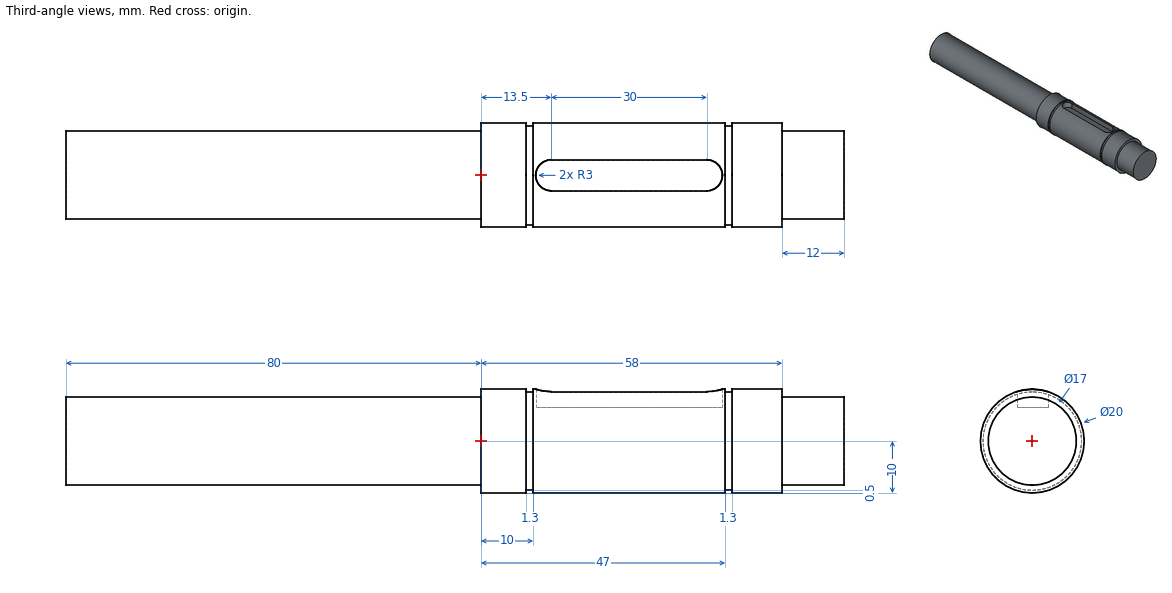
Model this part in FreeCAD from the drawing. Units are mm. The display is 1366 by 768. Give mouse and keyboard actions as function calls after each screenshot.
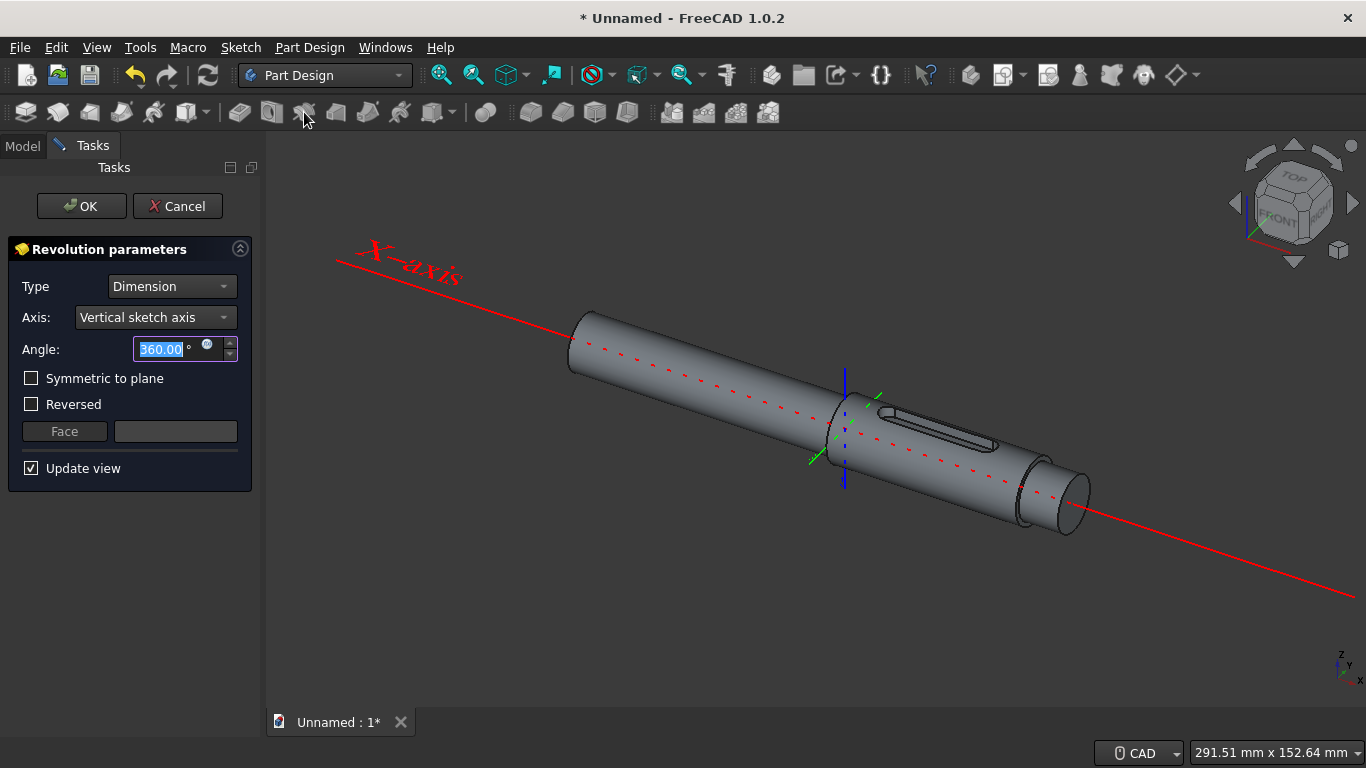
click(156, 318)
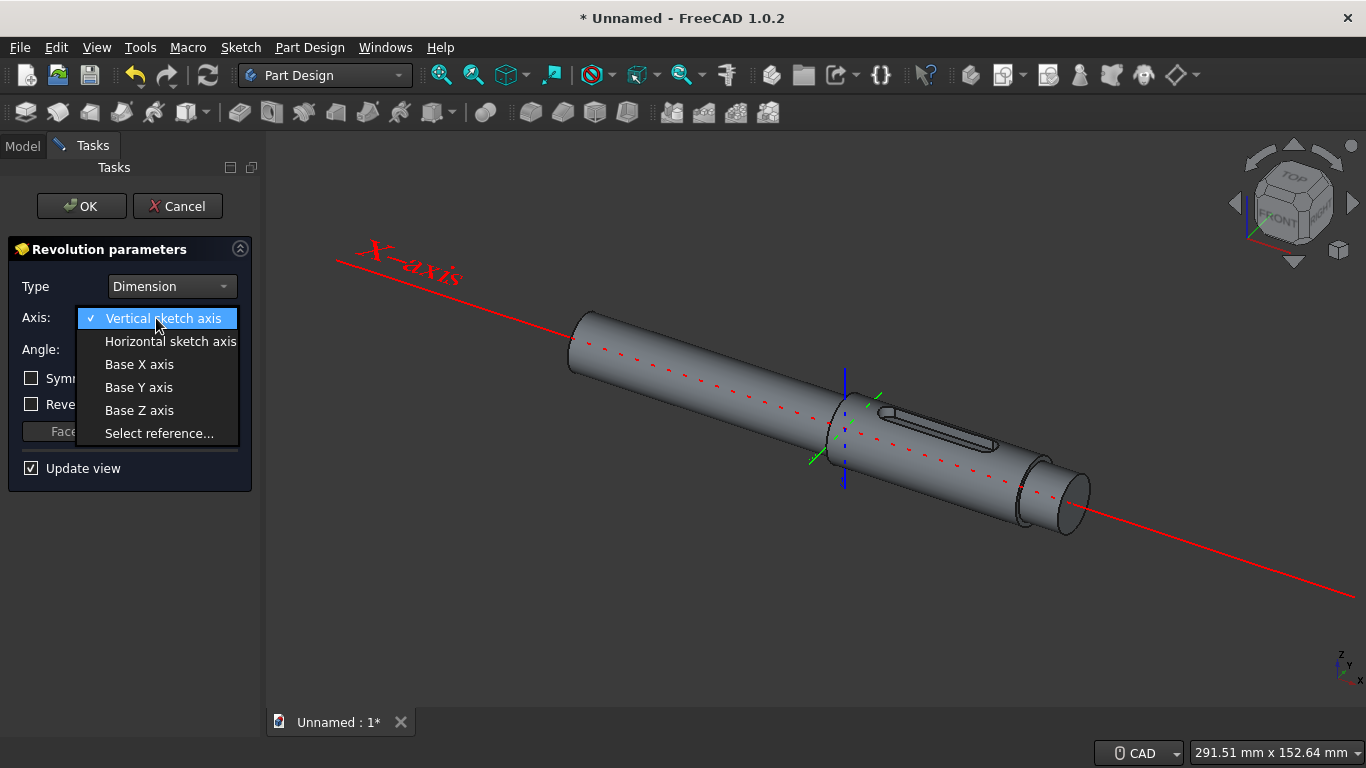
click(156, 342)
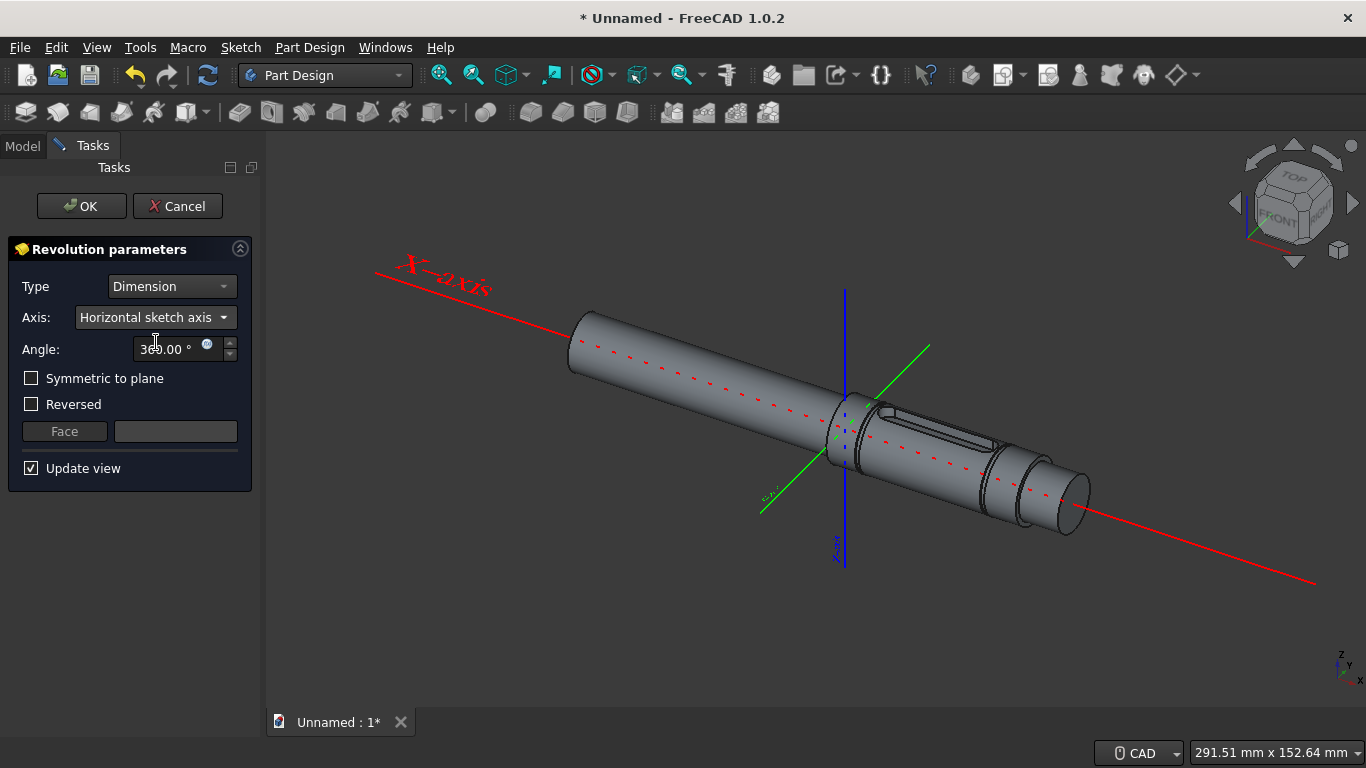
click(82, 206)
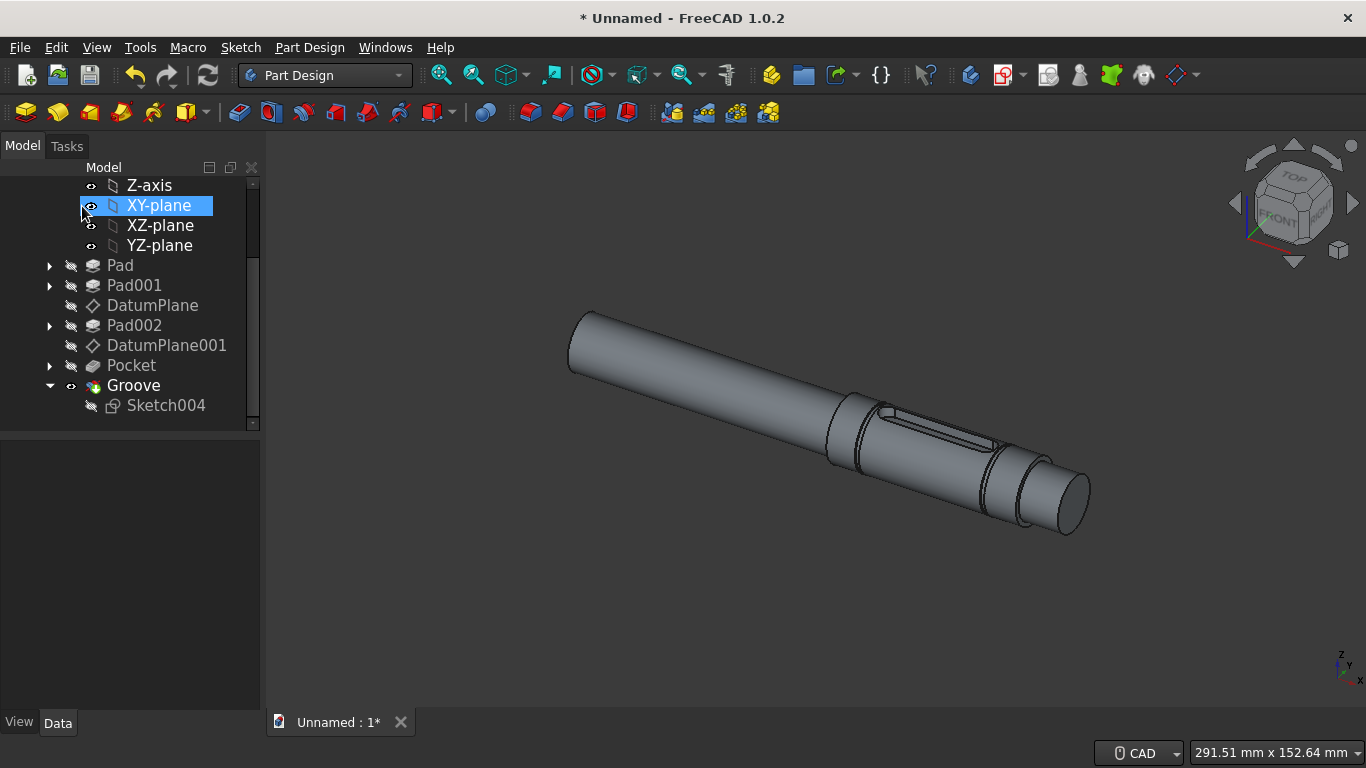
key(0)